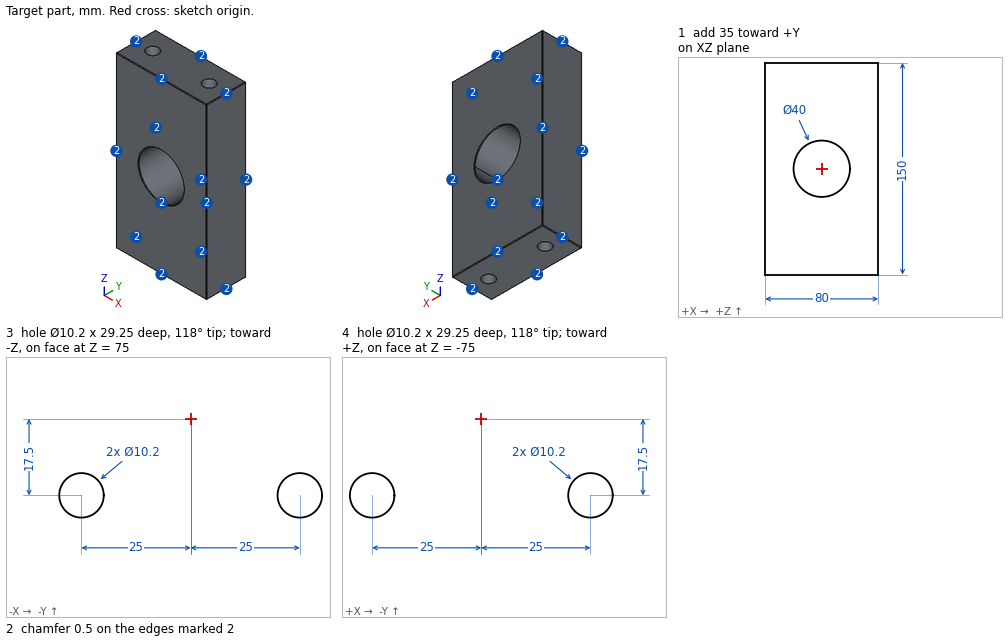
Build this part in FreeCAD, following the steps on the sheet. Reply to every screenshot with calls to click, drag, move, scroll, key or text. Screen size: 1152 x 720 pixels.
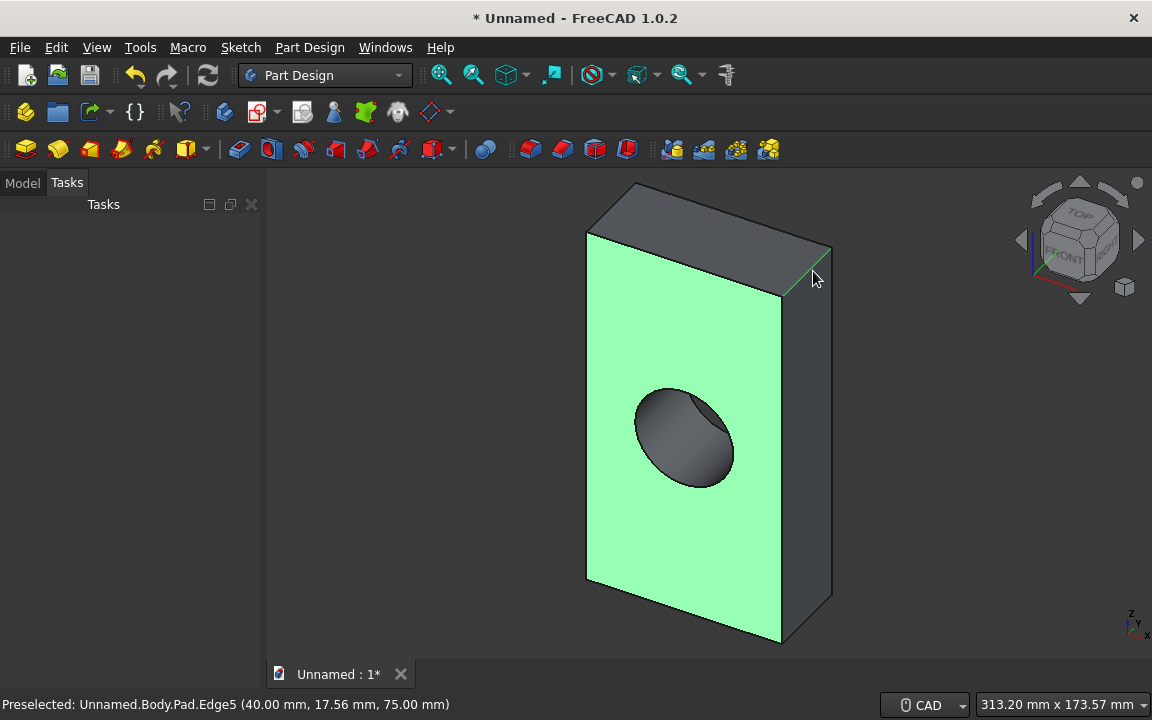
key(0)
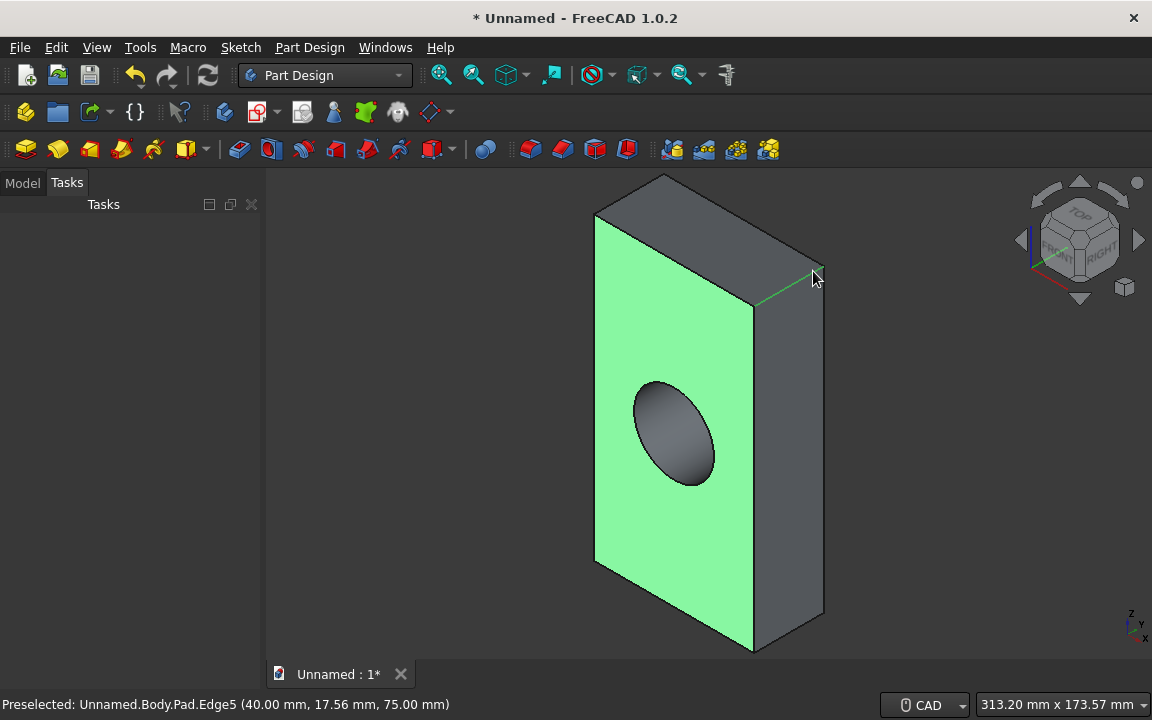
key(2)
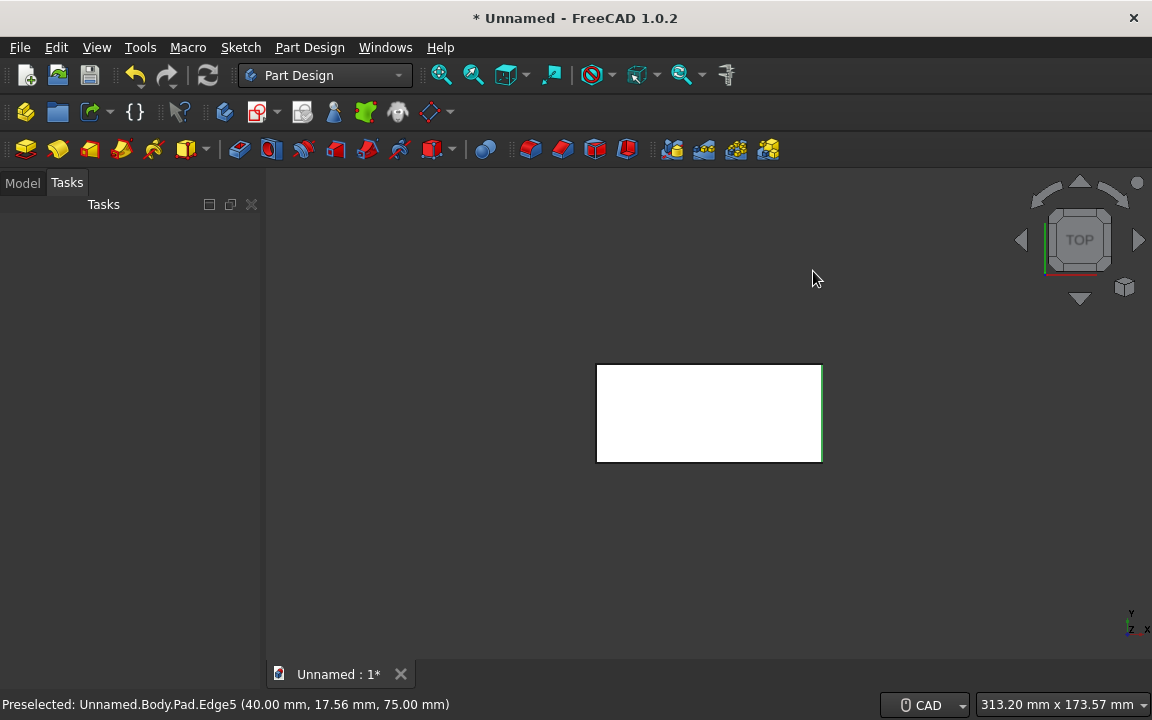
click(442, 76)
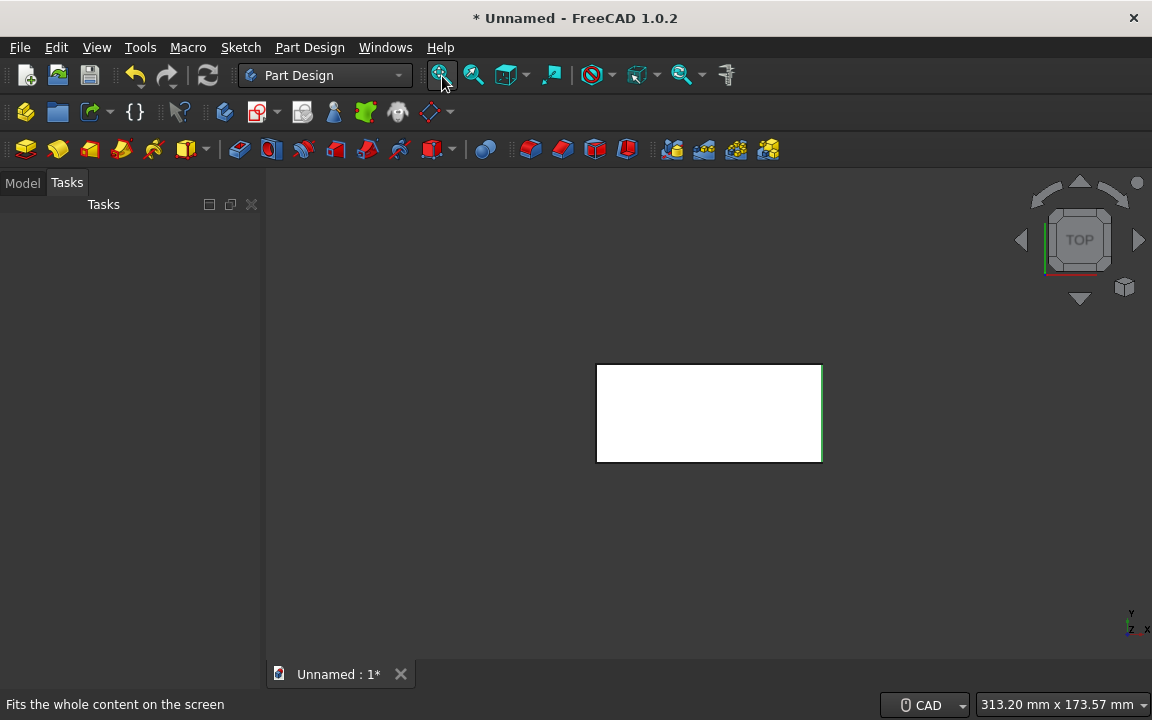
click(596, 412, ctrl)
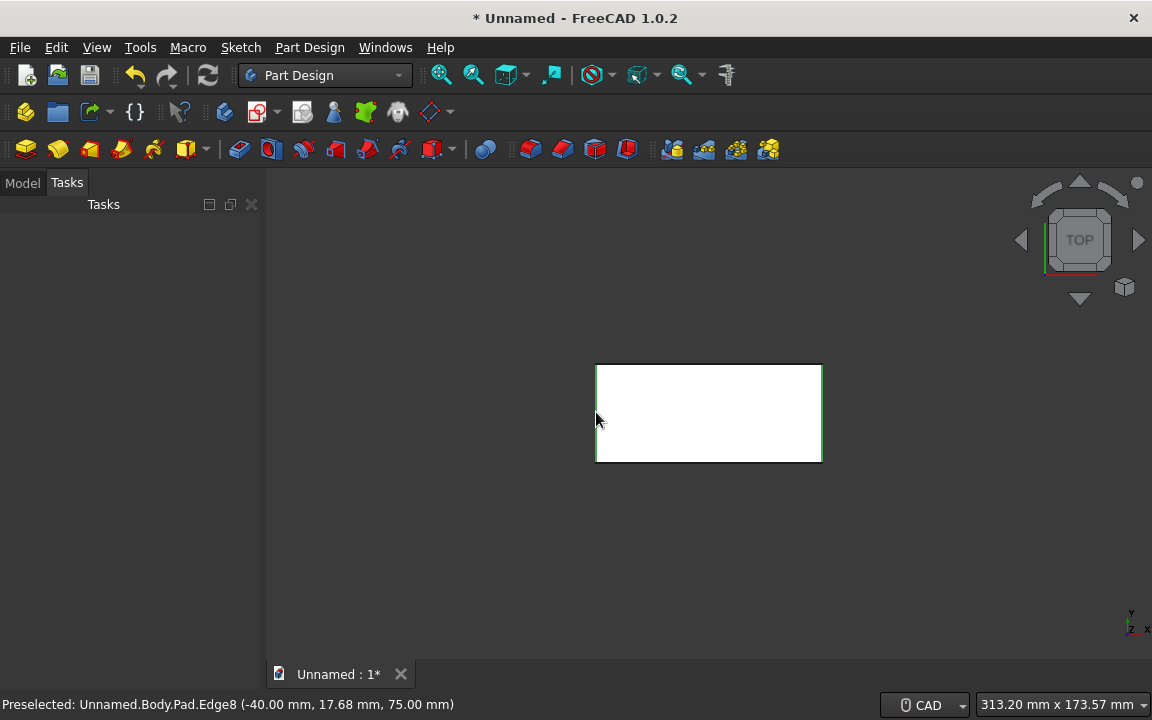
key(1)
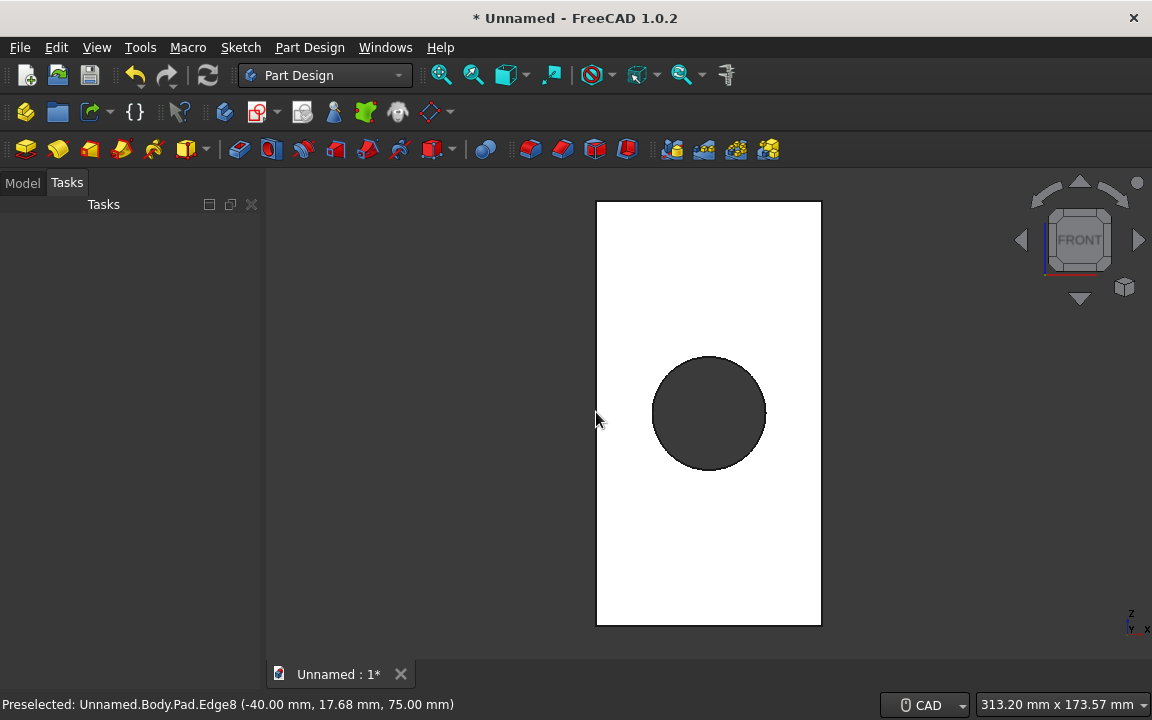
key(3)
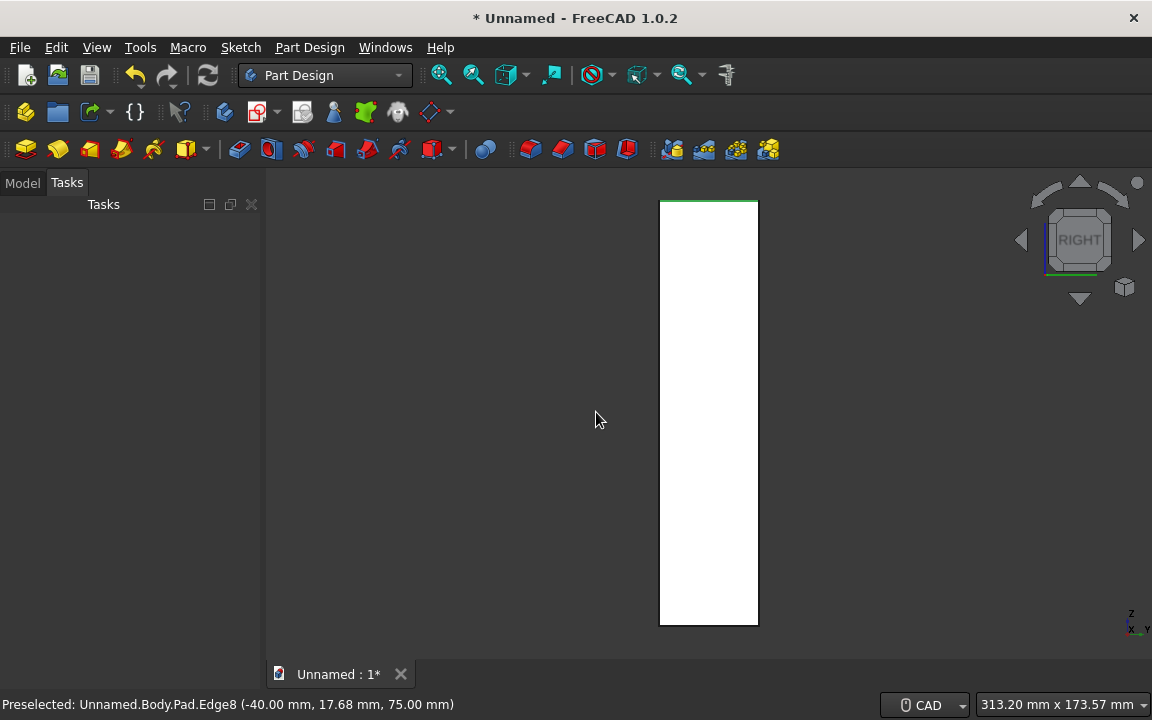
click(709, 625, ctrl)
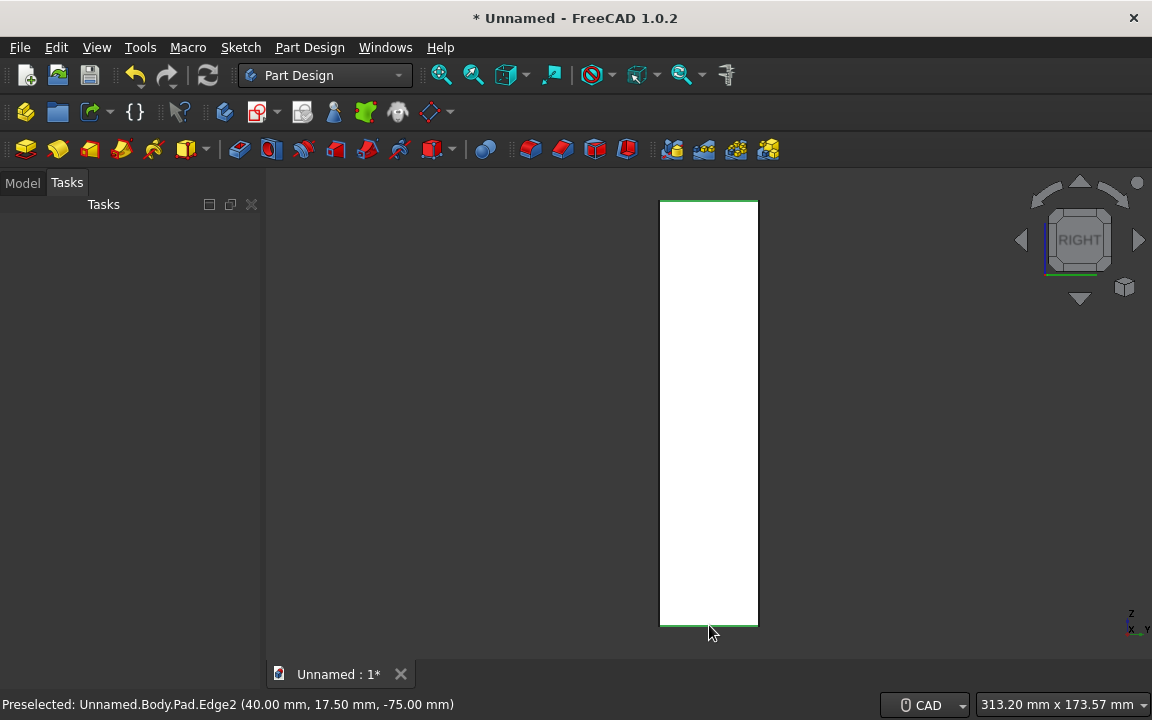
key(5)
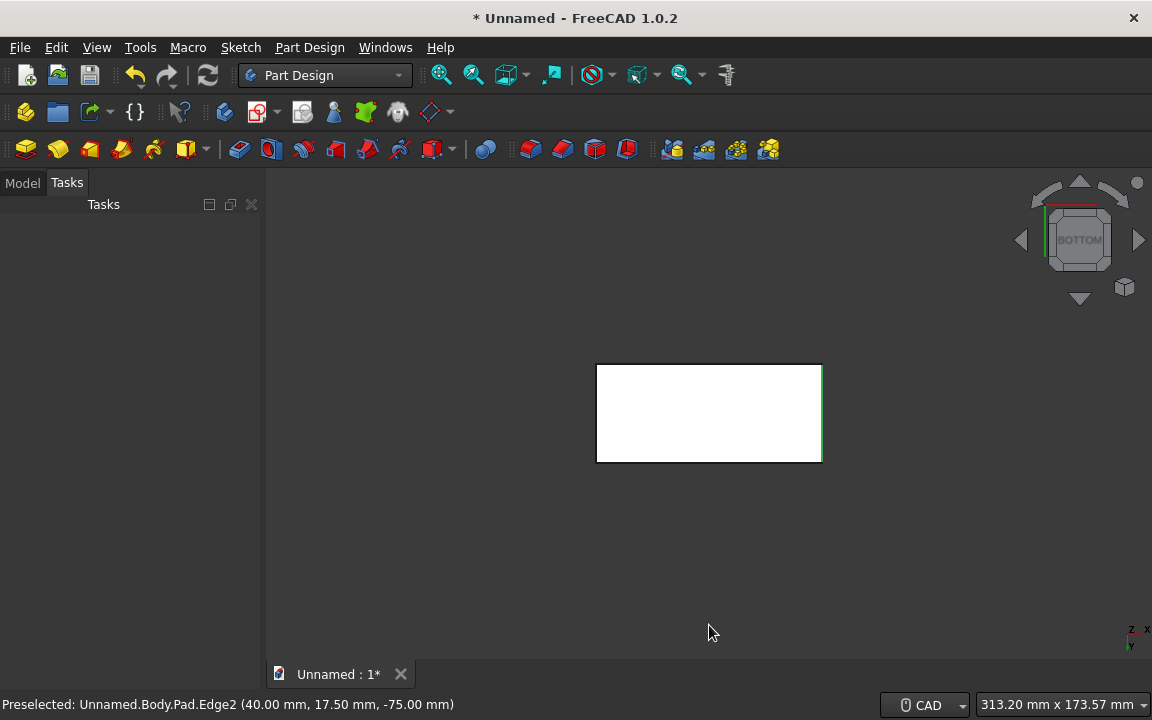
key(v)
key(f)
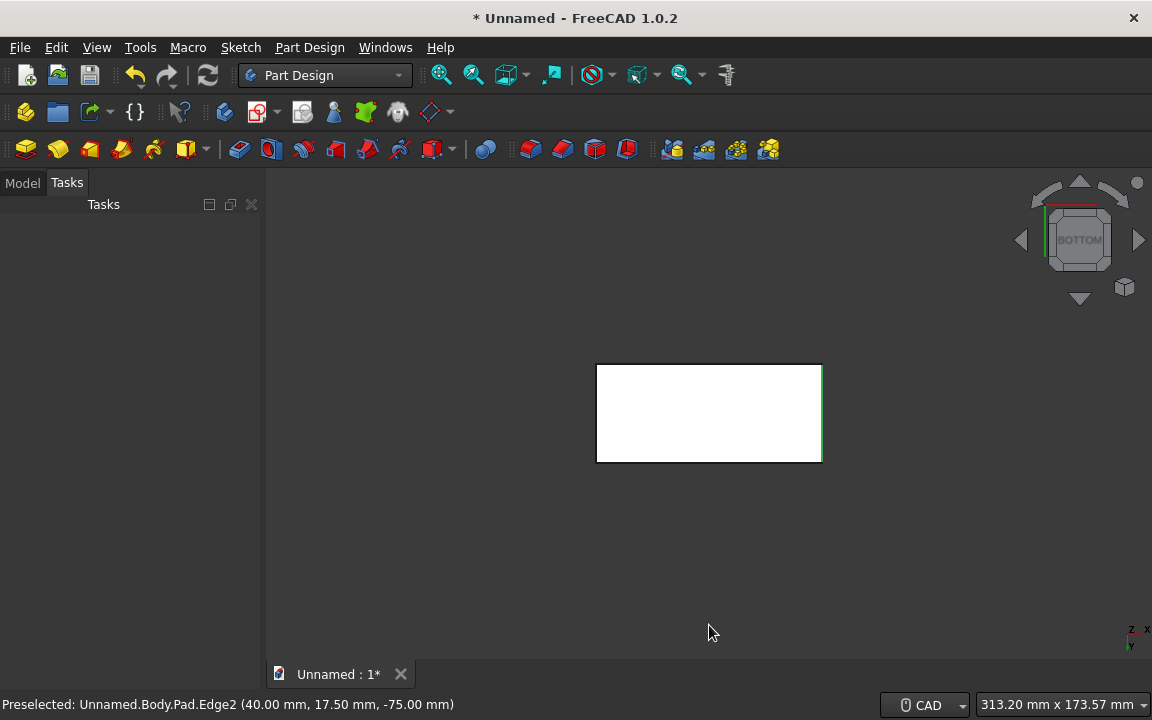
click(596, 412, ctrl)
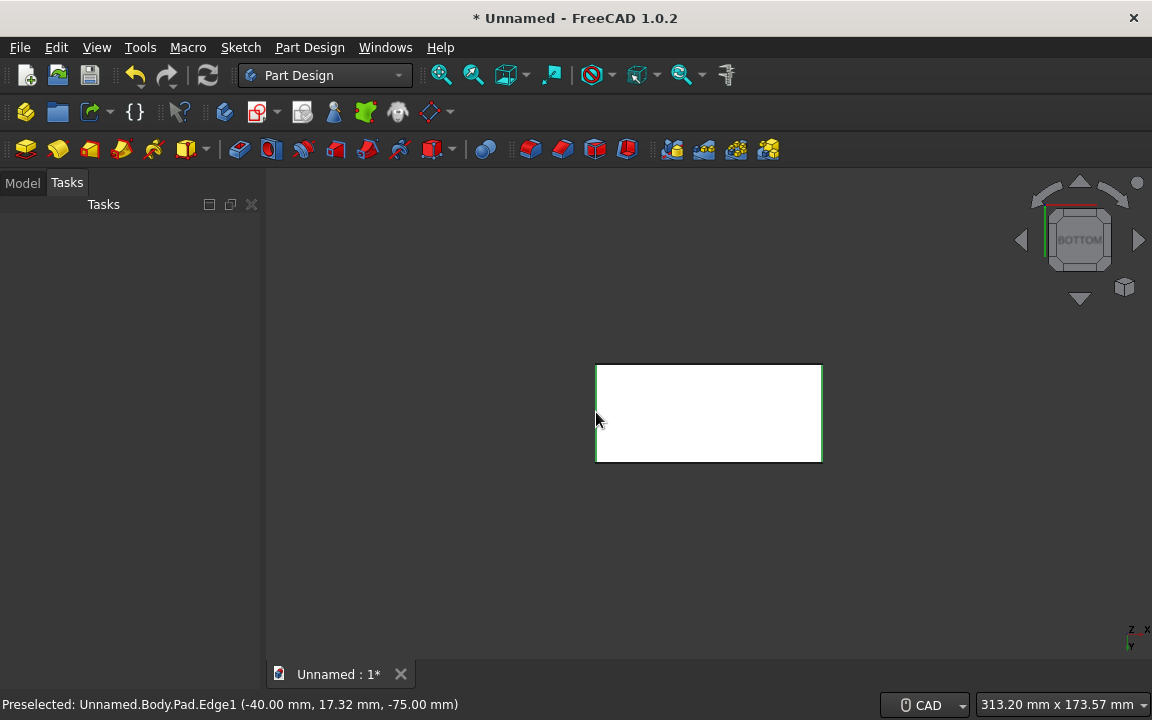
key(4)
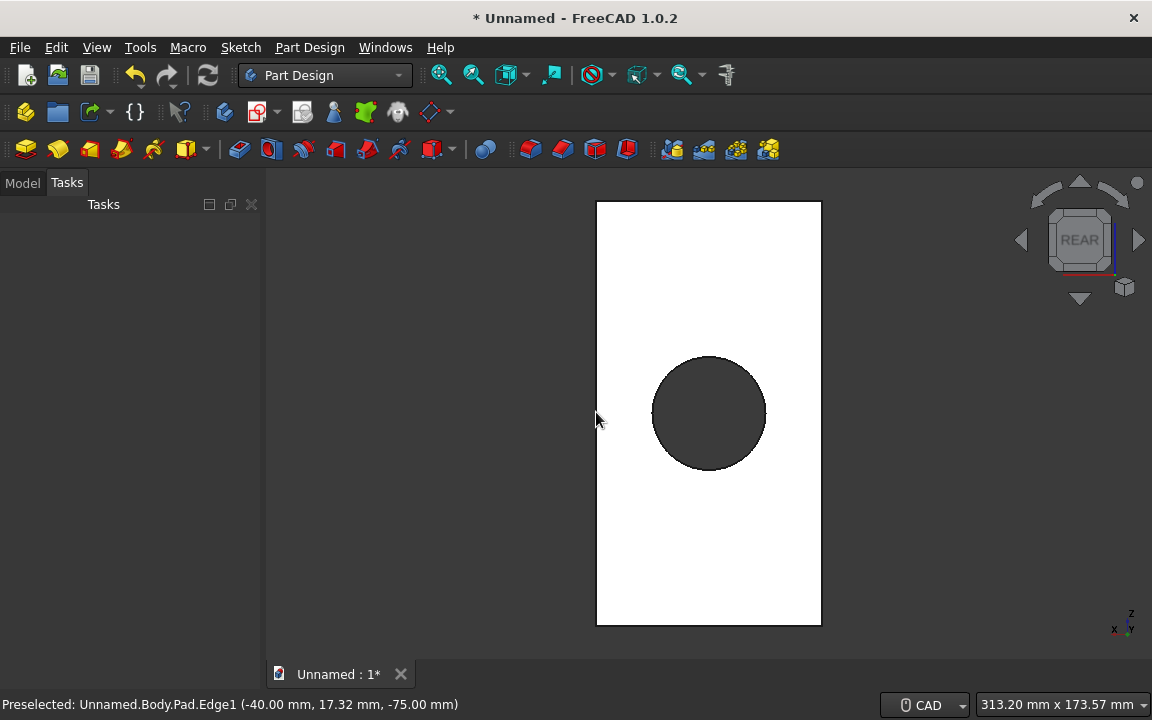
click(677, 291, ctrl)